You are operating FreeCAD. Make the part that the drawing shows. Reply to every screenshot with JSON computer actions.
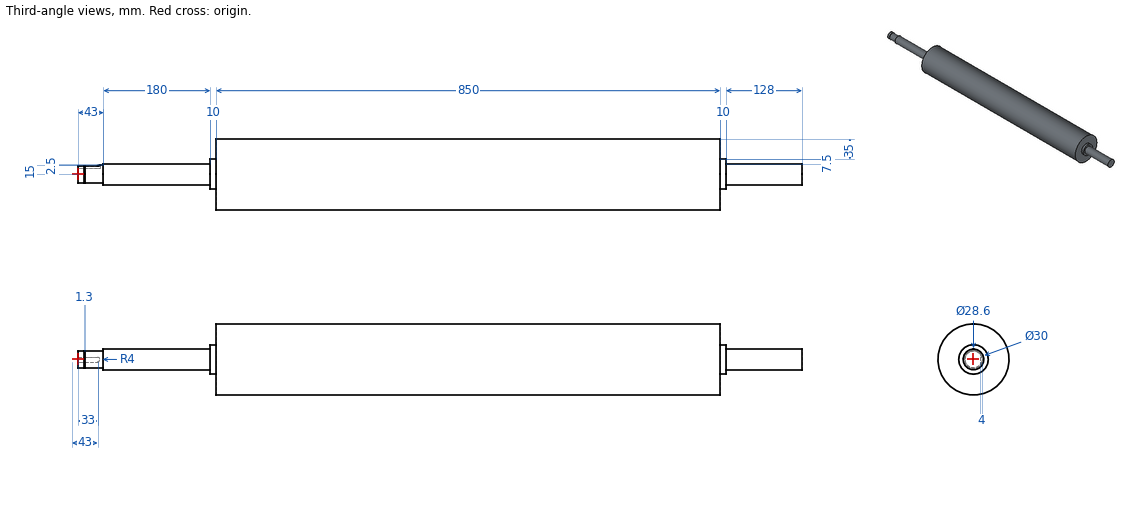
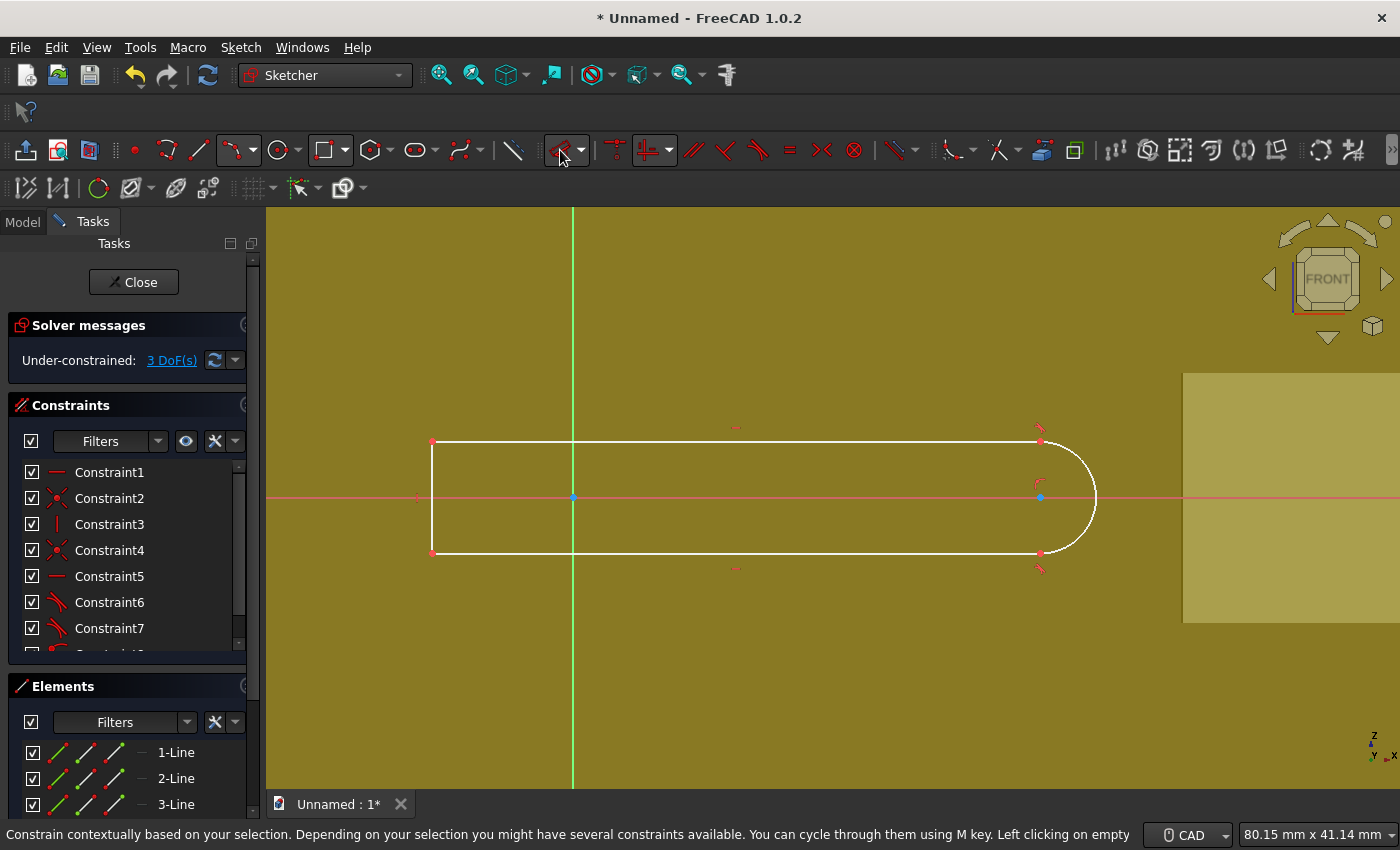
{"action": "left_click", "coordinate": [1085, 531]}
{"action": "left_click", "coordinate": [1111, 550]}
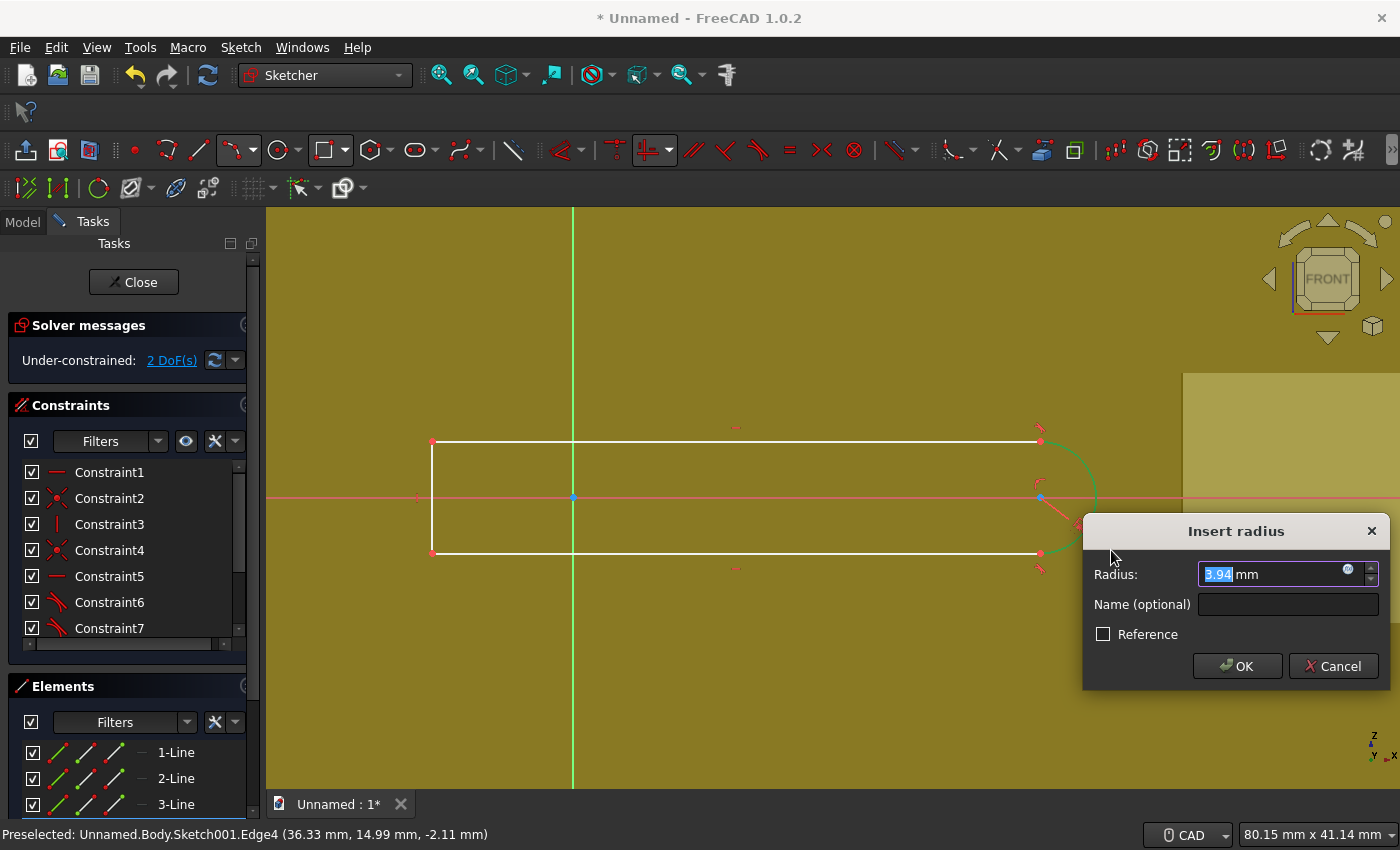
{"action": "type", "text": "4"}
{"action": "key", "text": "Return"}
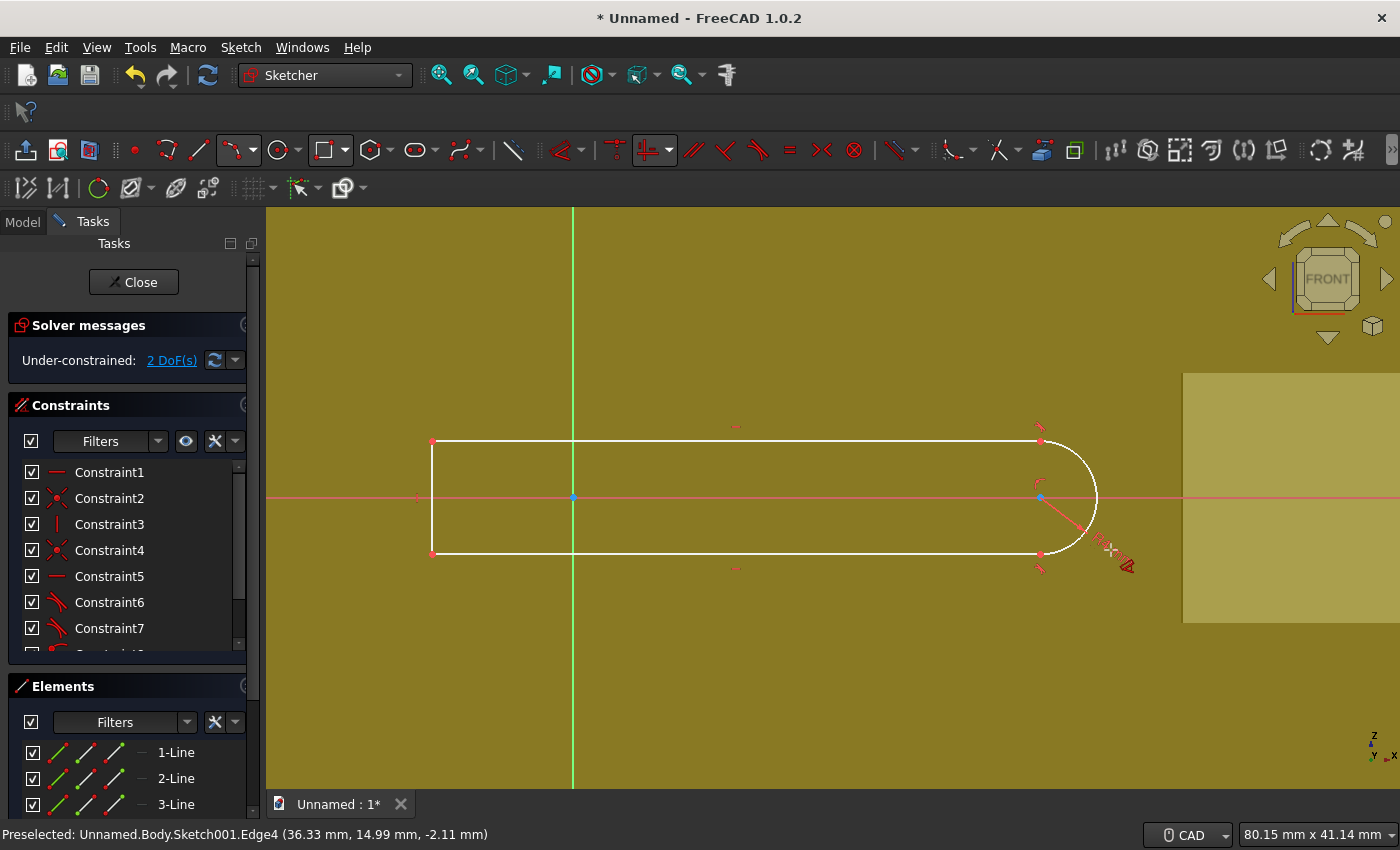
{"action": "left_click", "coordinate": [858, 554]}
{"action": "left_click", "coordinate": [736, 588]}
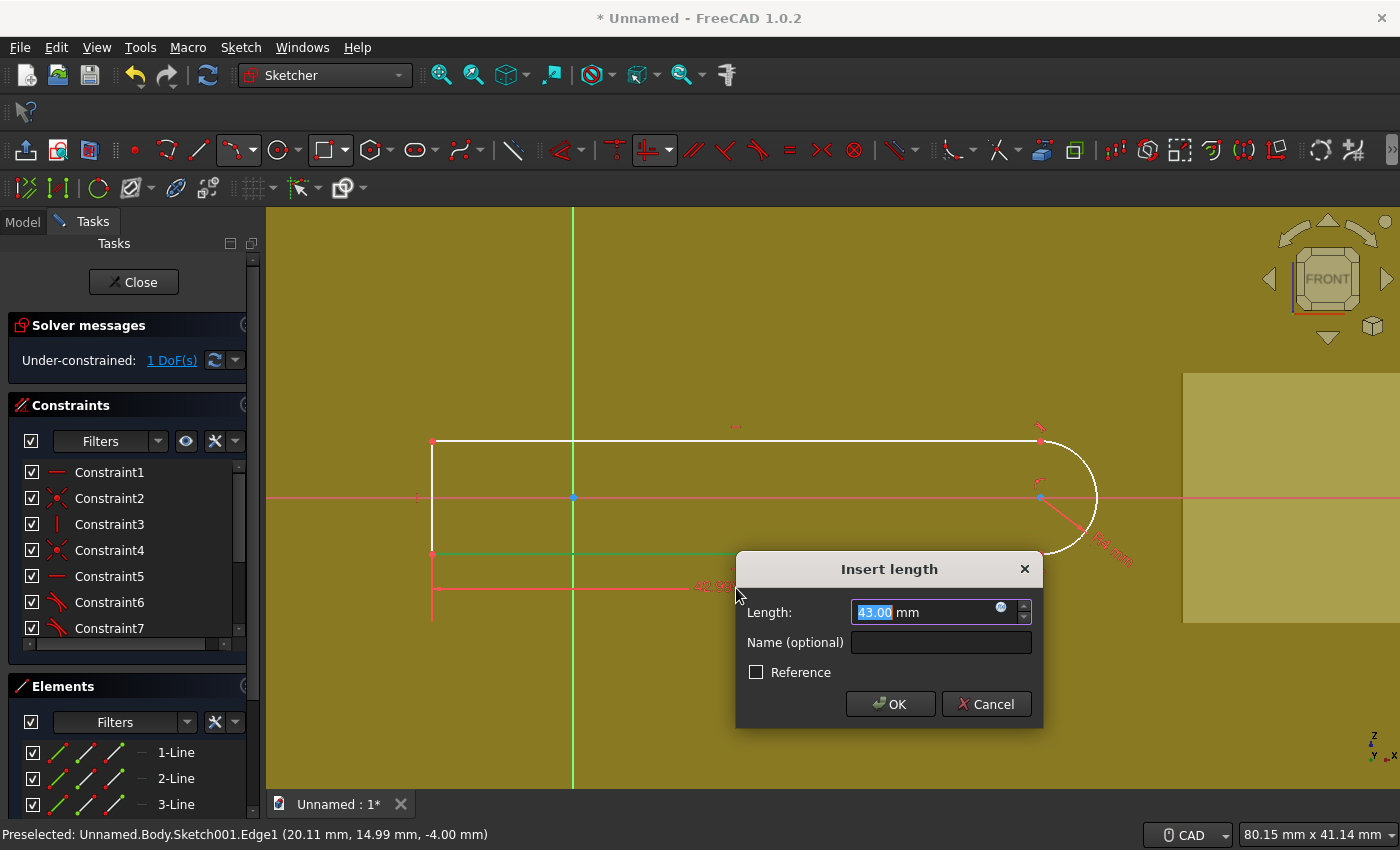
{"action": "type", "text": "43"}
{"action": "key", "text": "Return"}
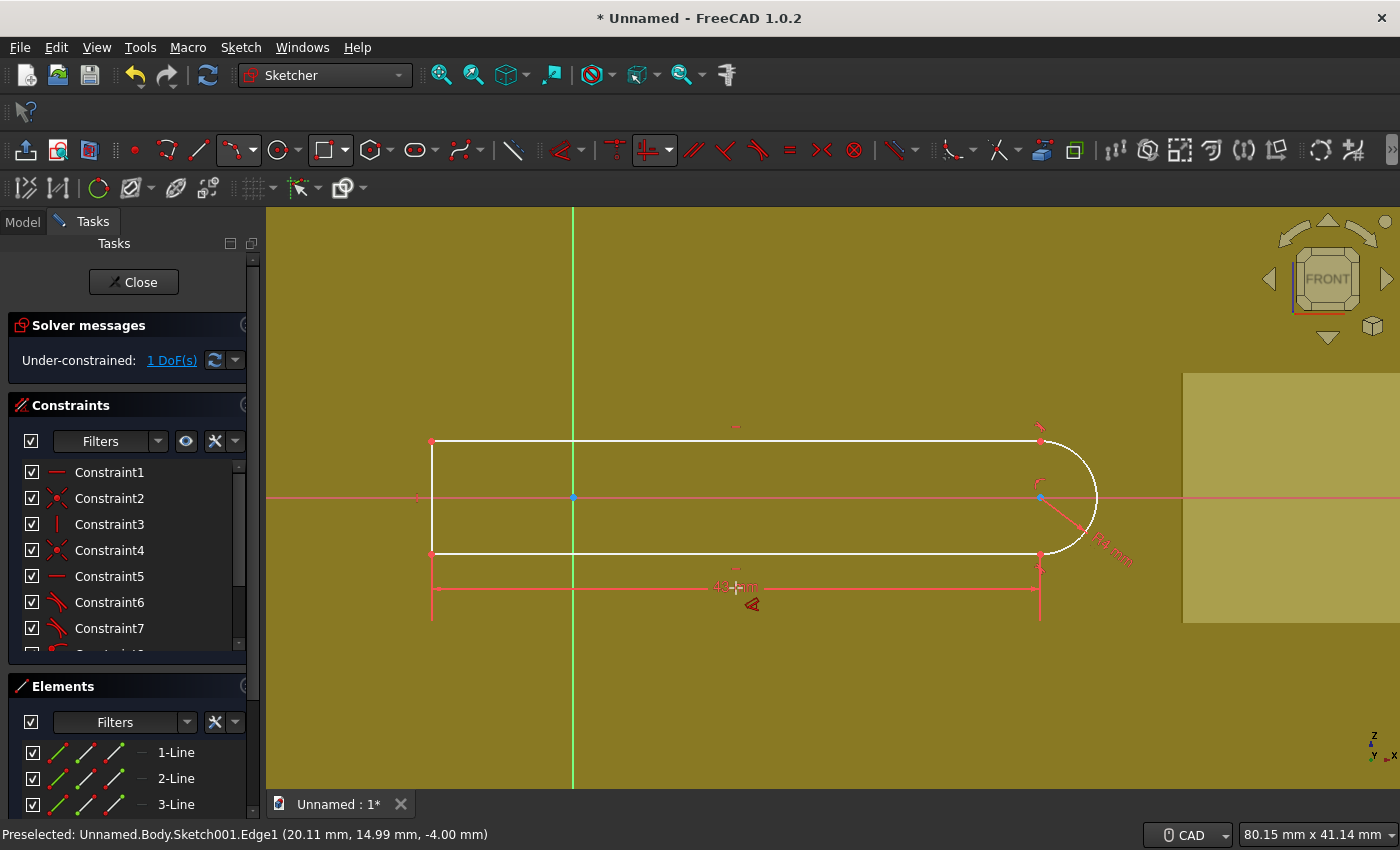
{"action": "left_click", "coordinate": [1040, 554]}
{"action": "left_click", "coordinate": [807, 588]}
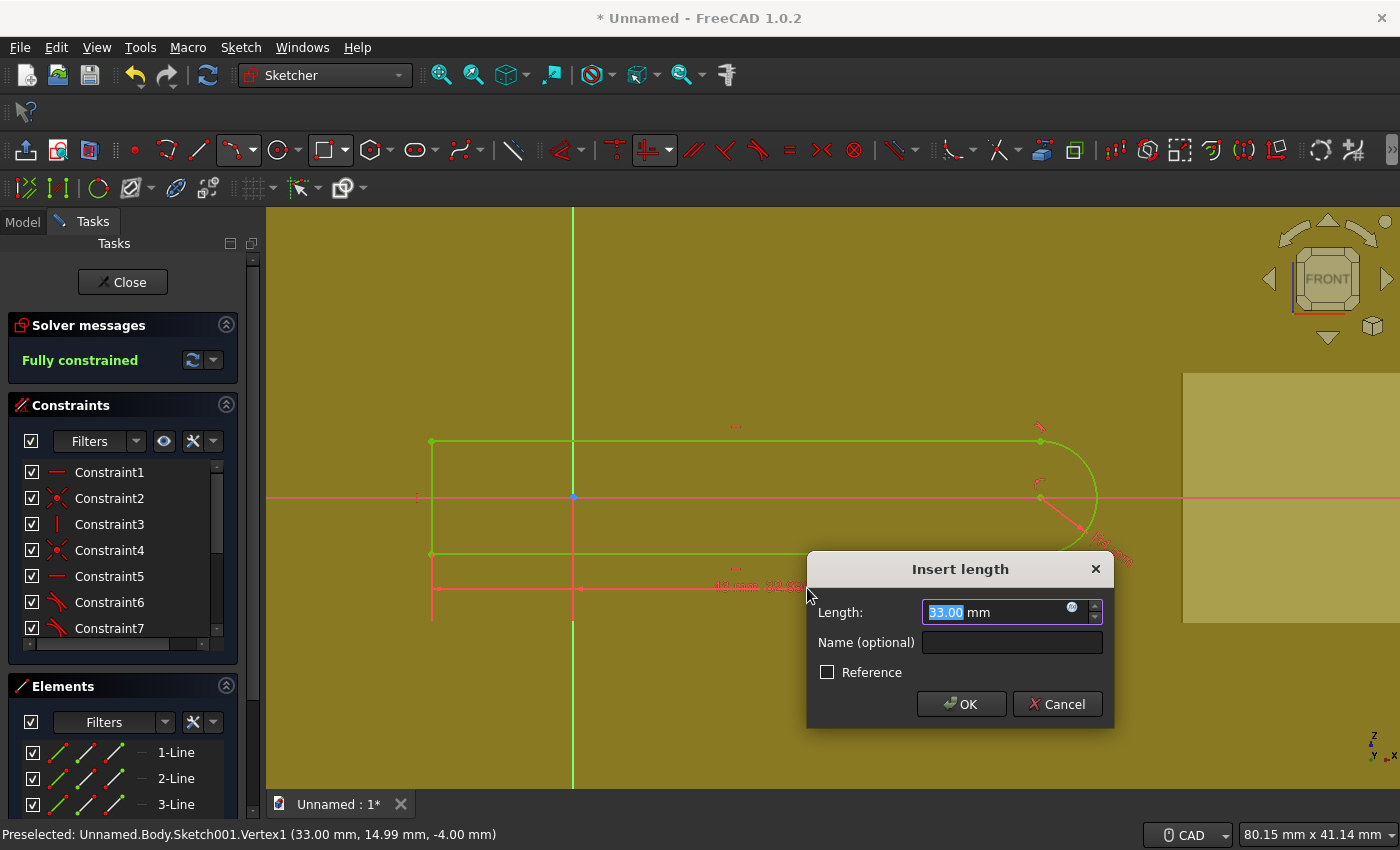
{"action": "type", "text": "33"}
{"action": "key", "text": "Return"}
{"action": "key", "text": "Escape"}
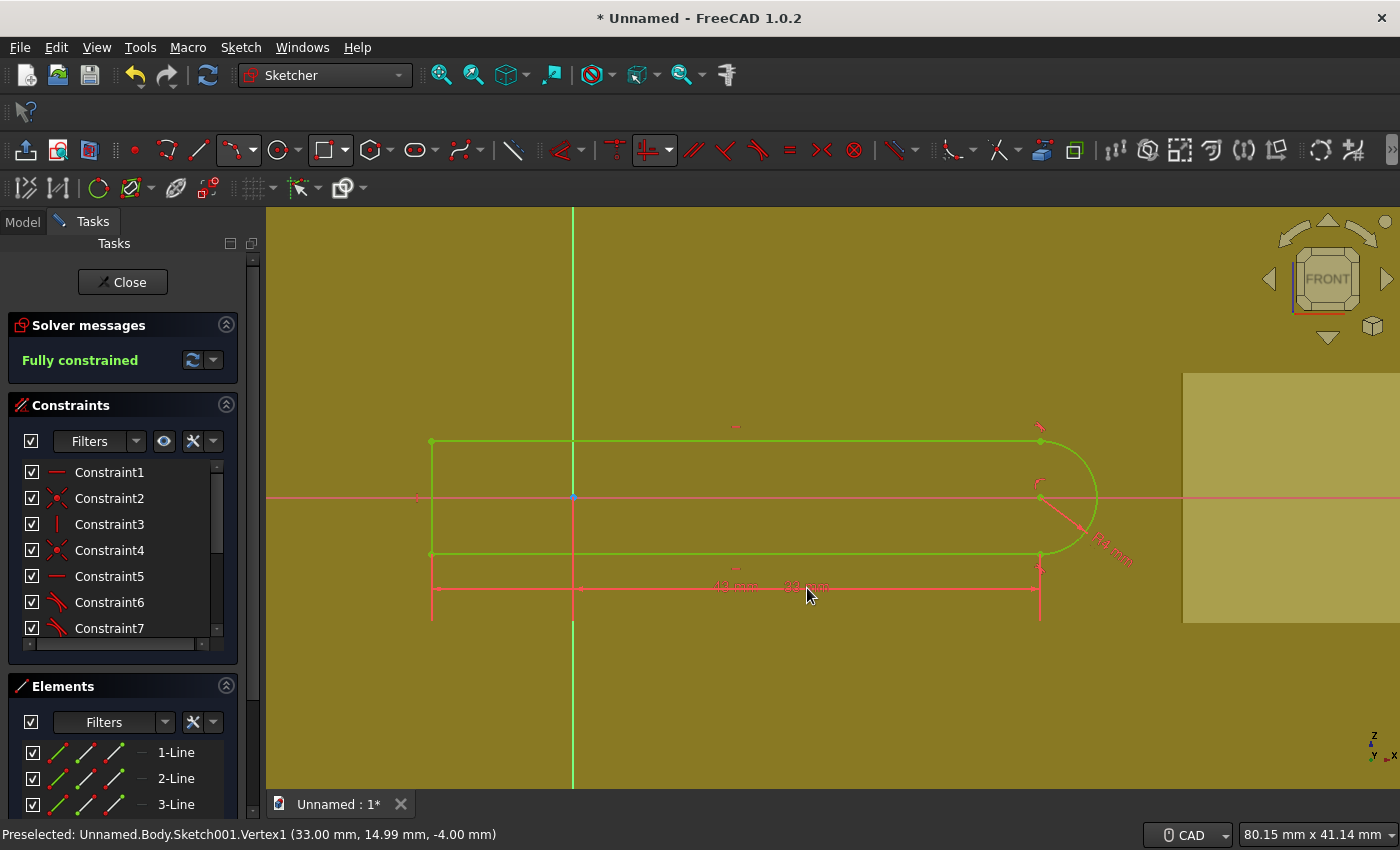
{"action": "left_click", "coordinate": [123, 282]}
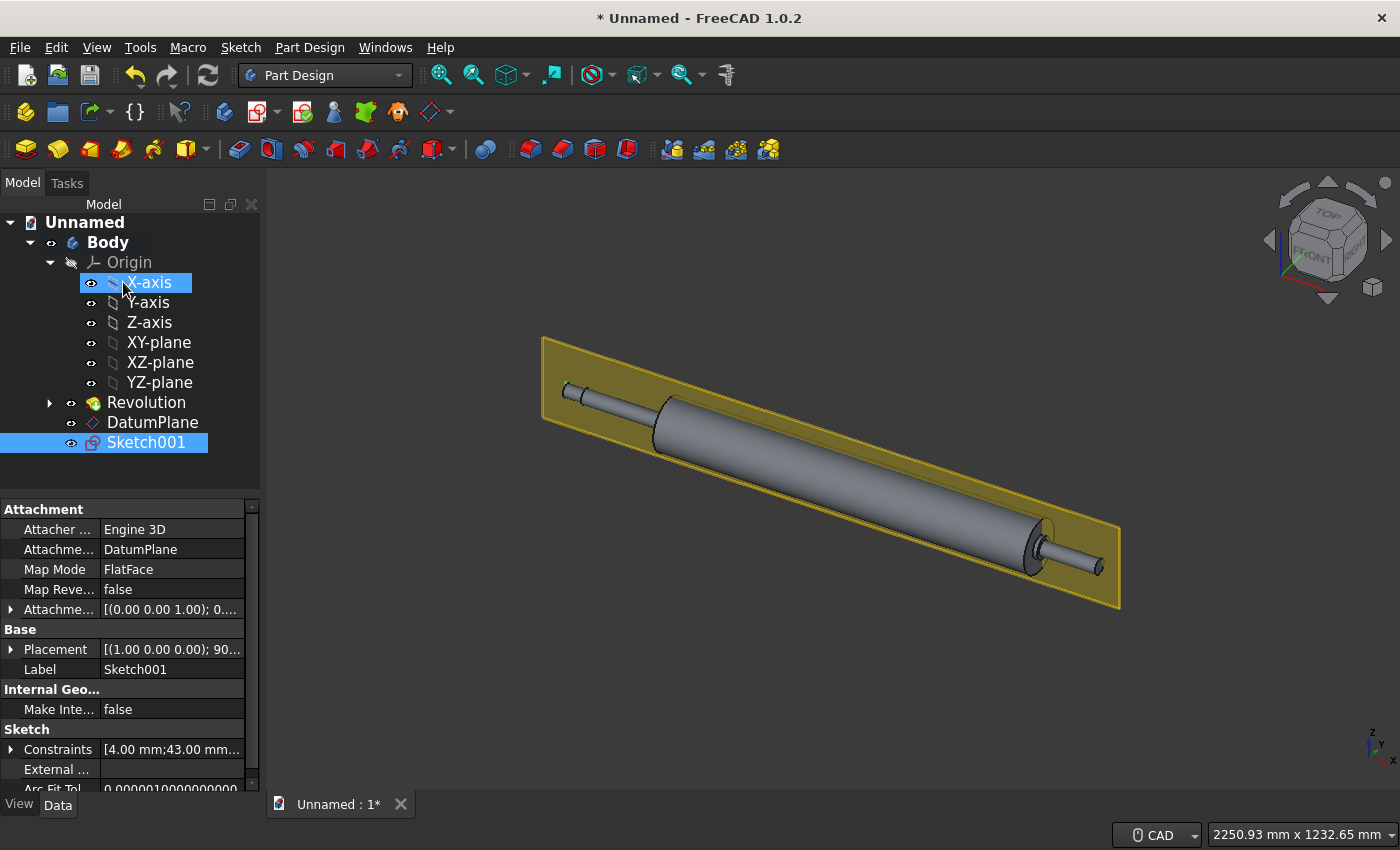
{"action": "left_click", "coordinate": [240, 150]}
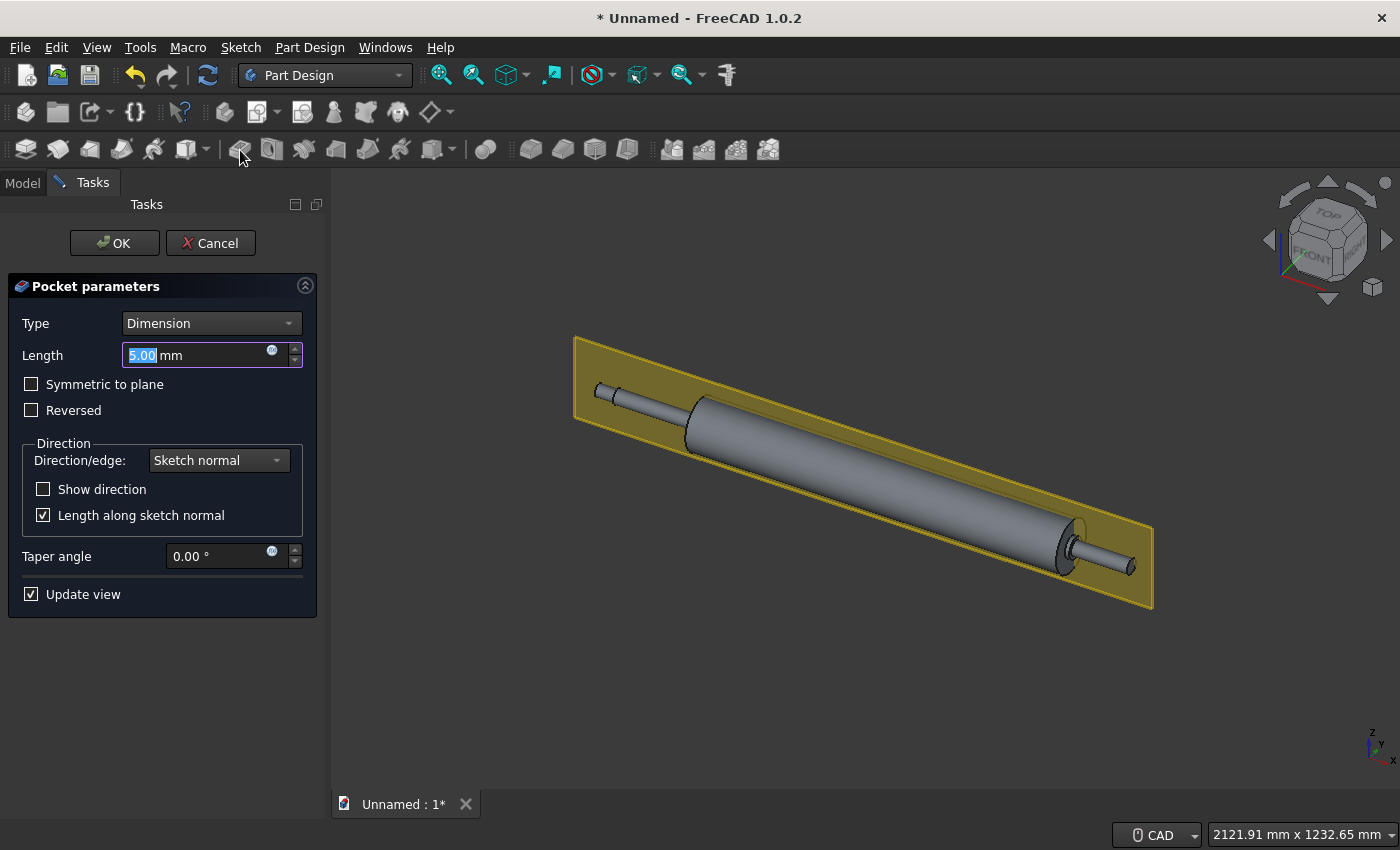
{"action": "type", "text": "4"}
{"action": "key", "text": "Tab"}